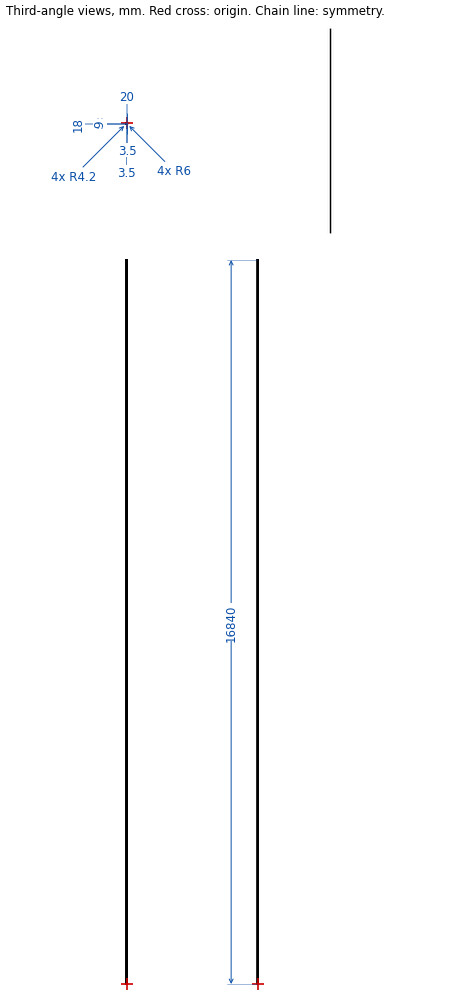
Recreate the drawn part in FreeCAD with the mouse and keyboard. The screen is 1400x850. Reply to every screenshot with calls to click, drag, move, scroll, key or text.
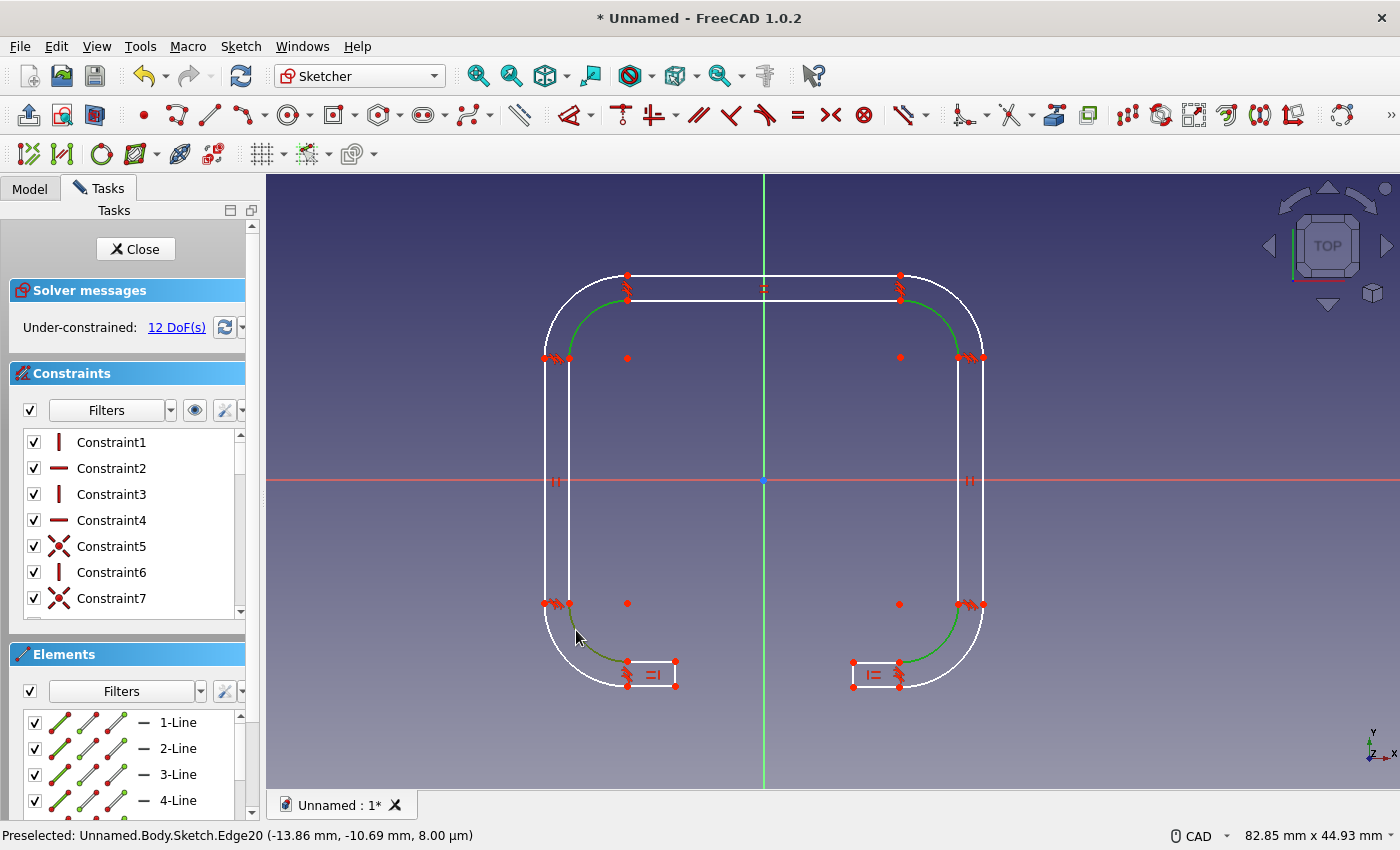
click(798, 116)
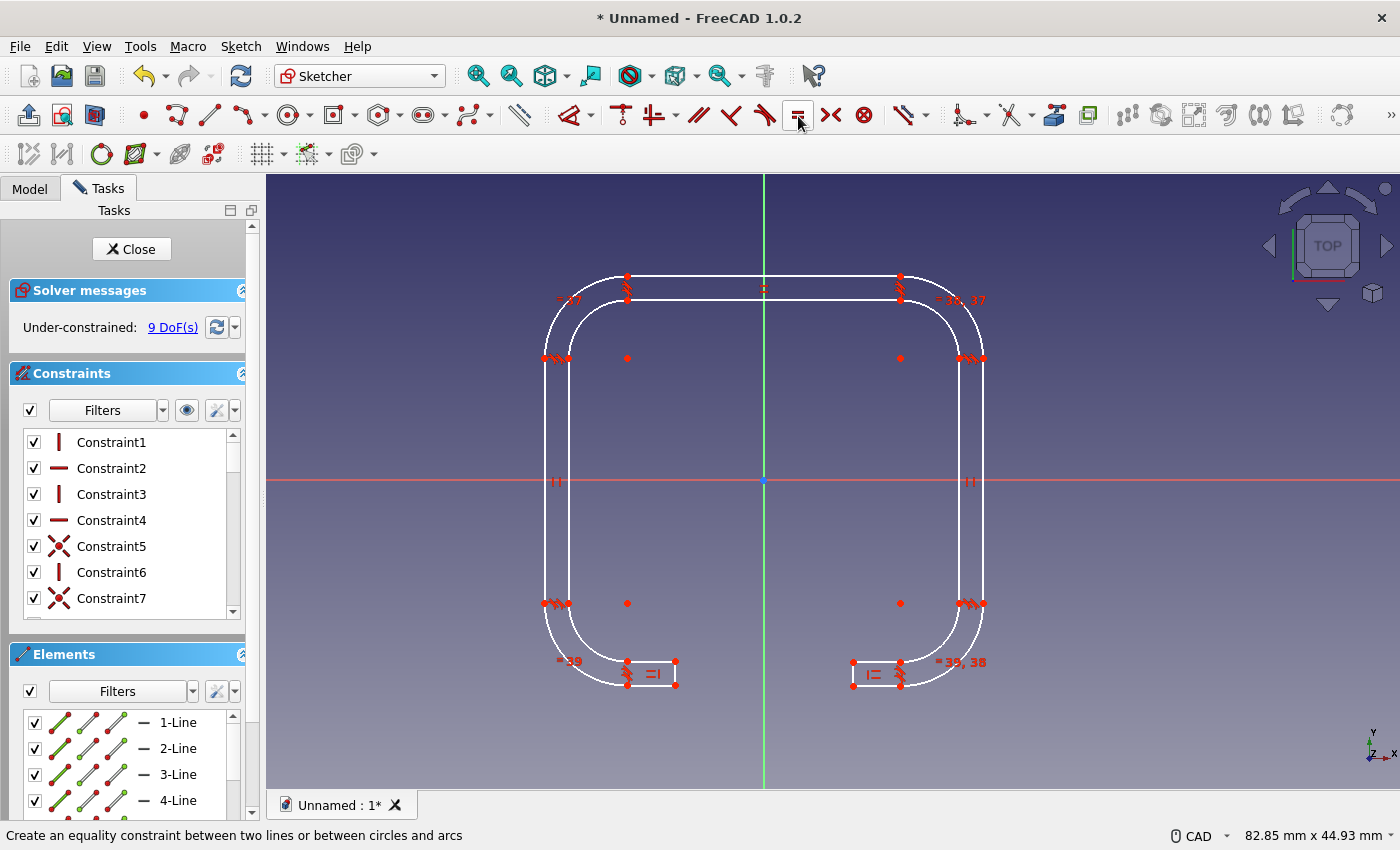
click(901, 604)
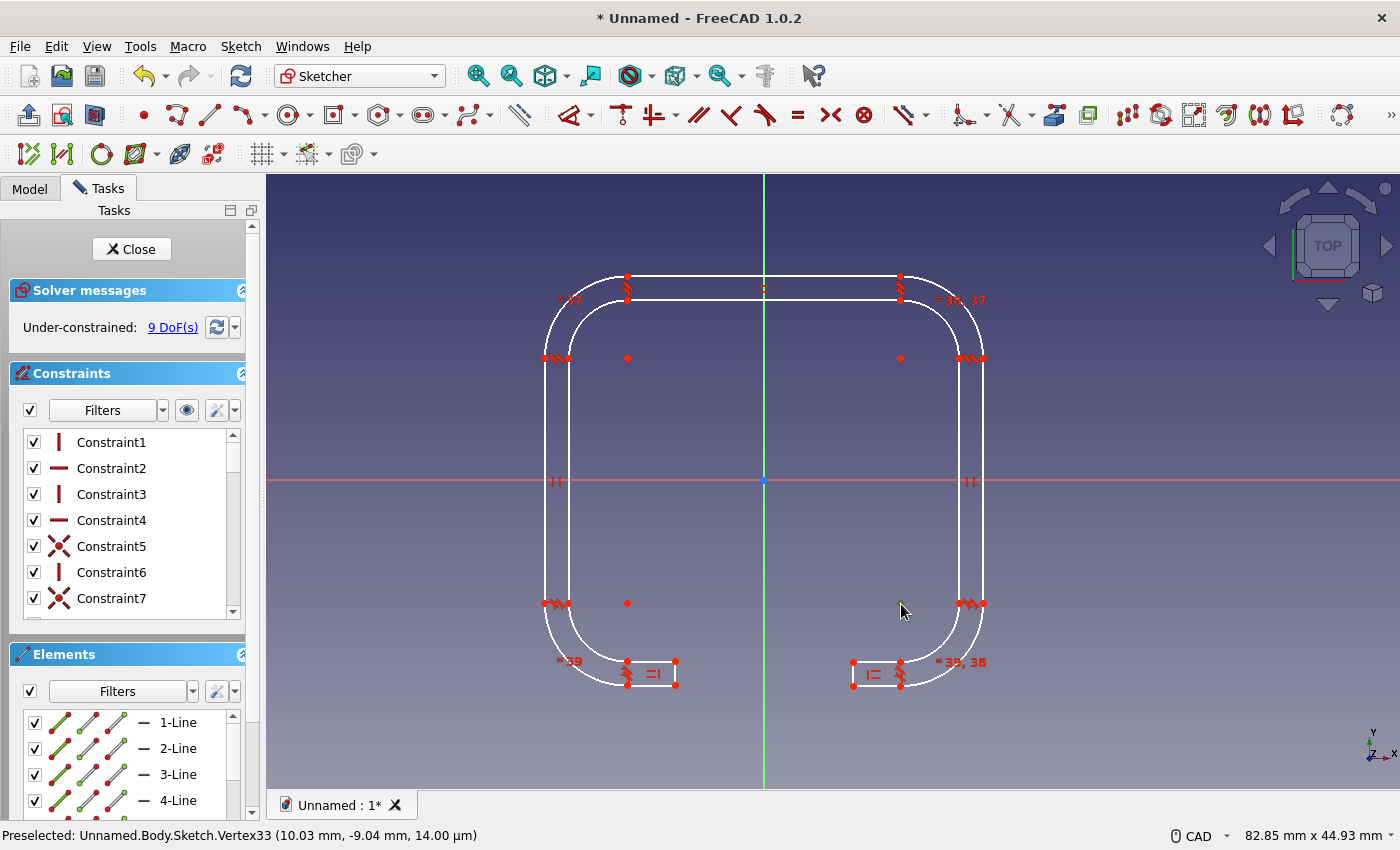
click(627, 603)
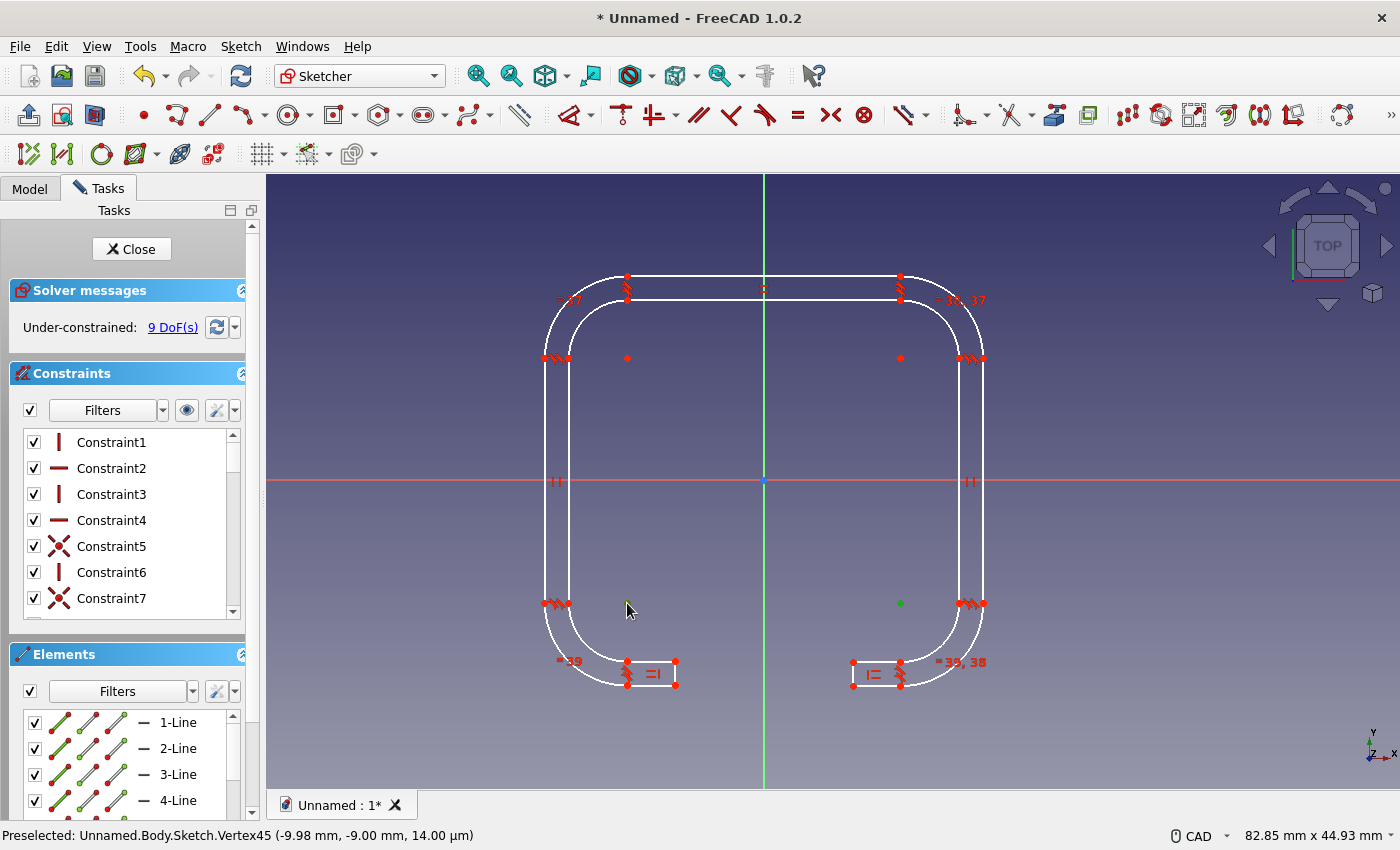
click(764, 721)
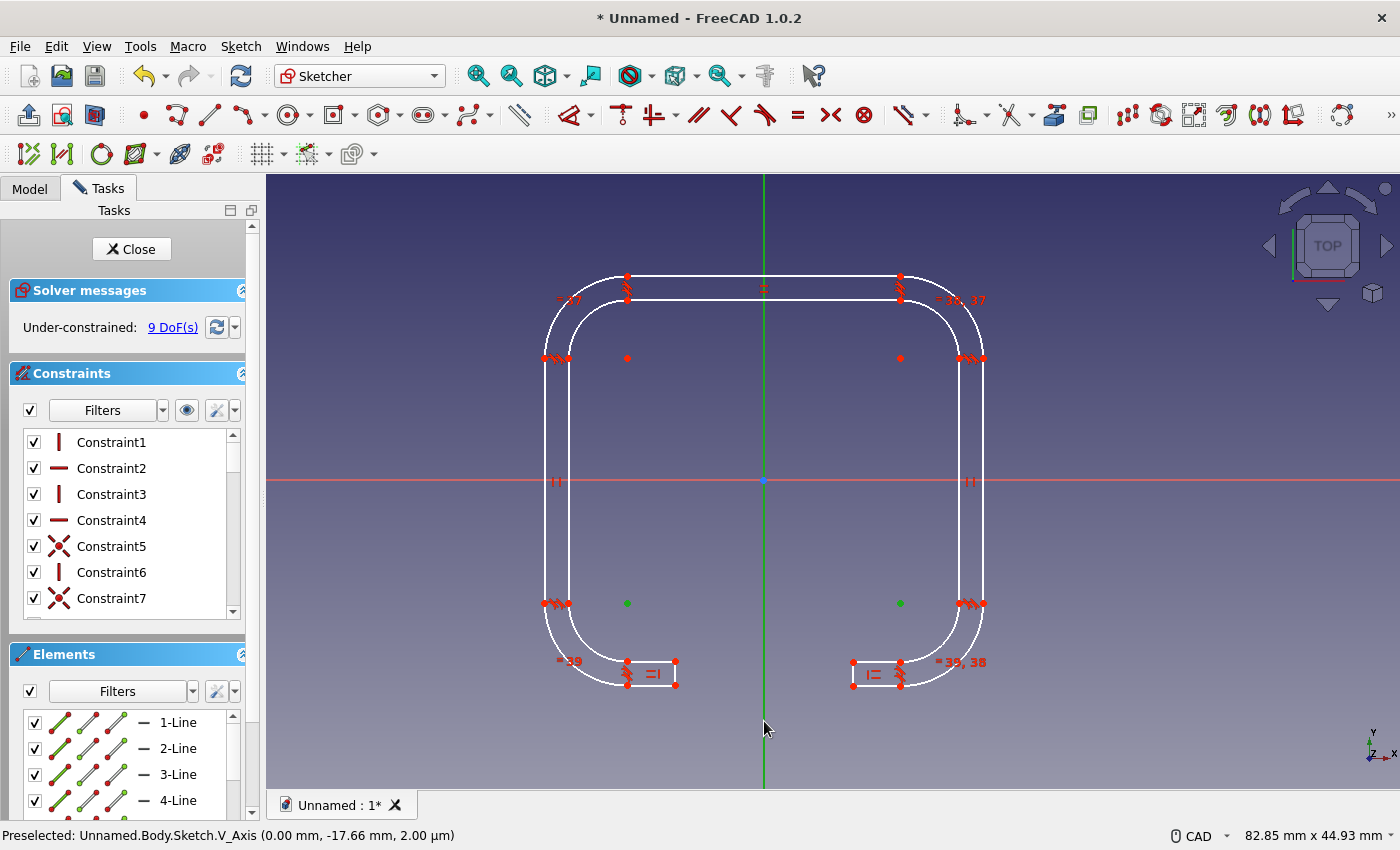
click(831, 116)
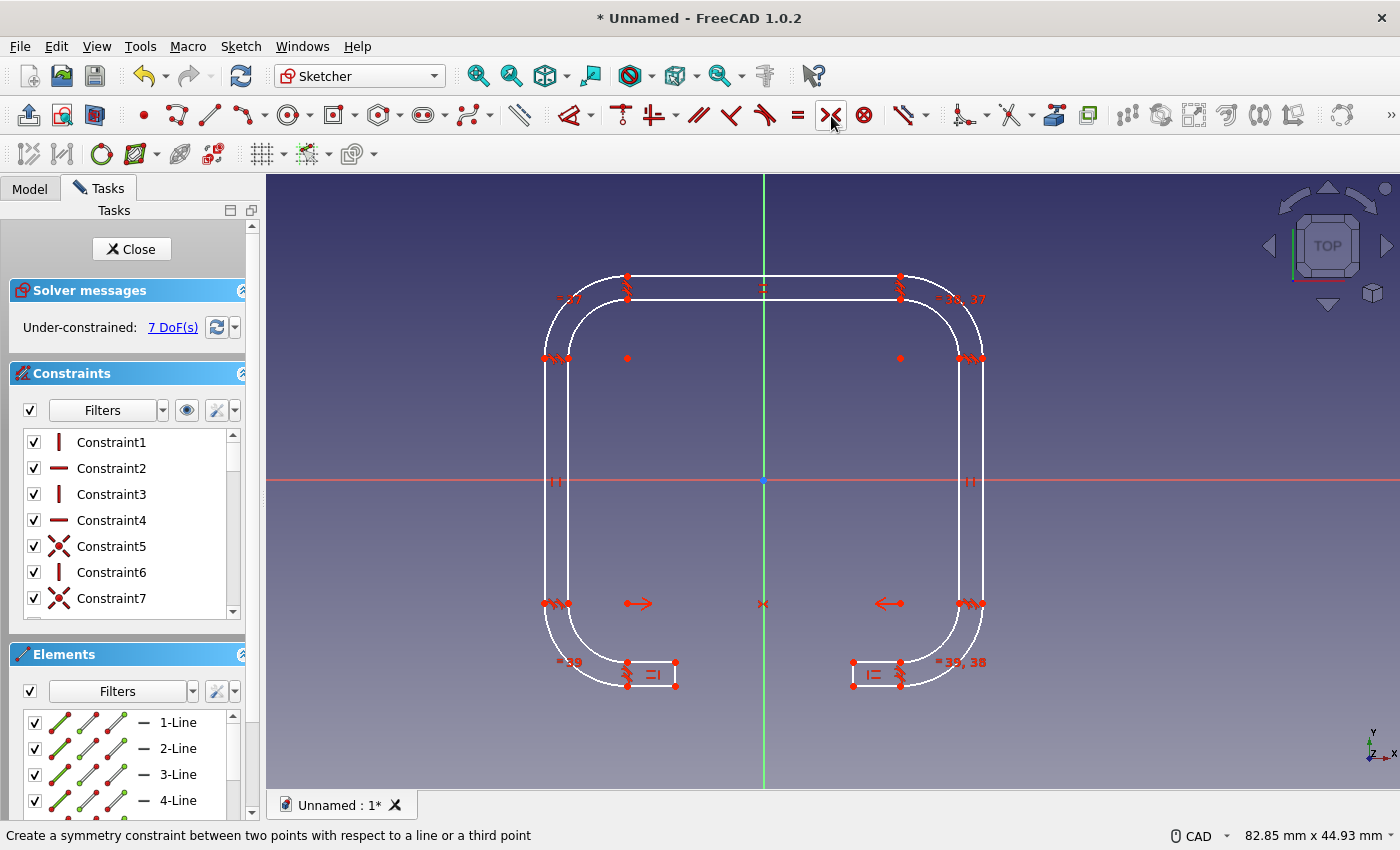
click(568, 116)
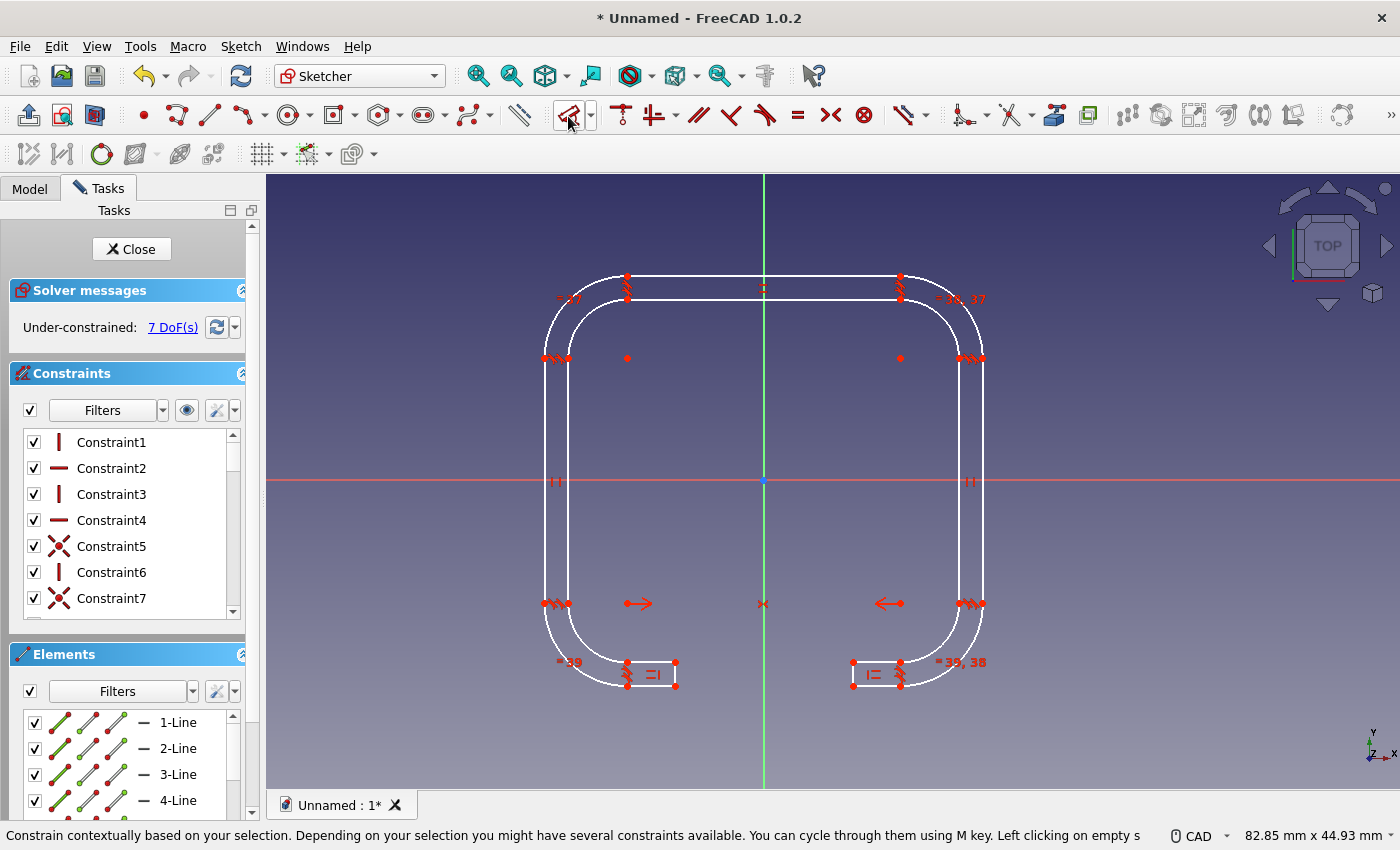
click(600, 306)
click(708, 317)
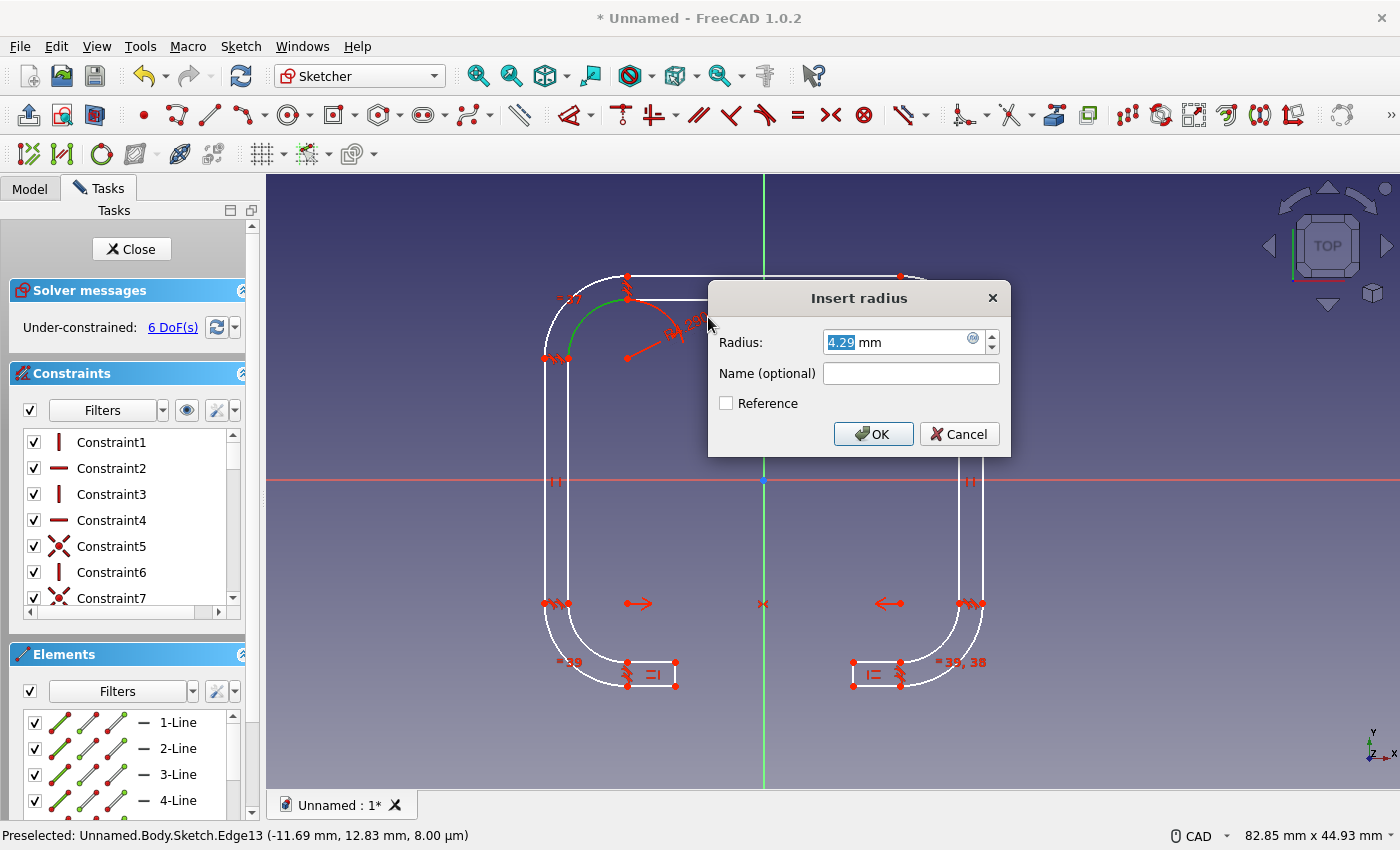
text(4.2)
key(Return)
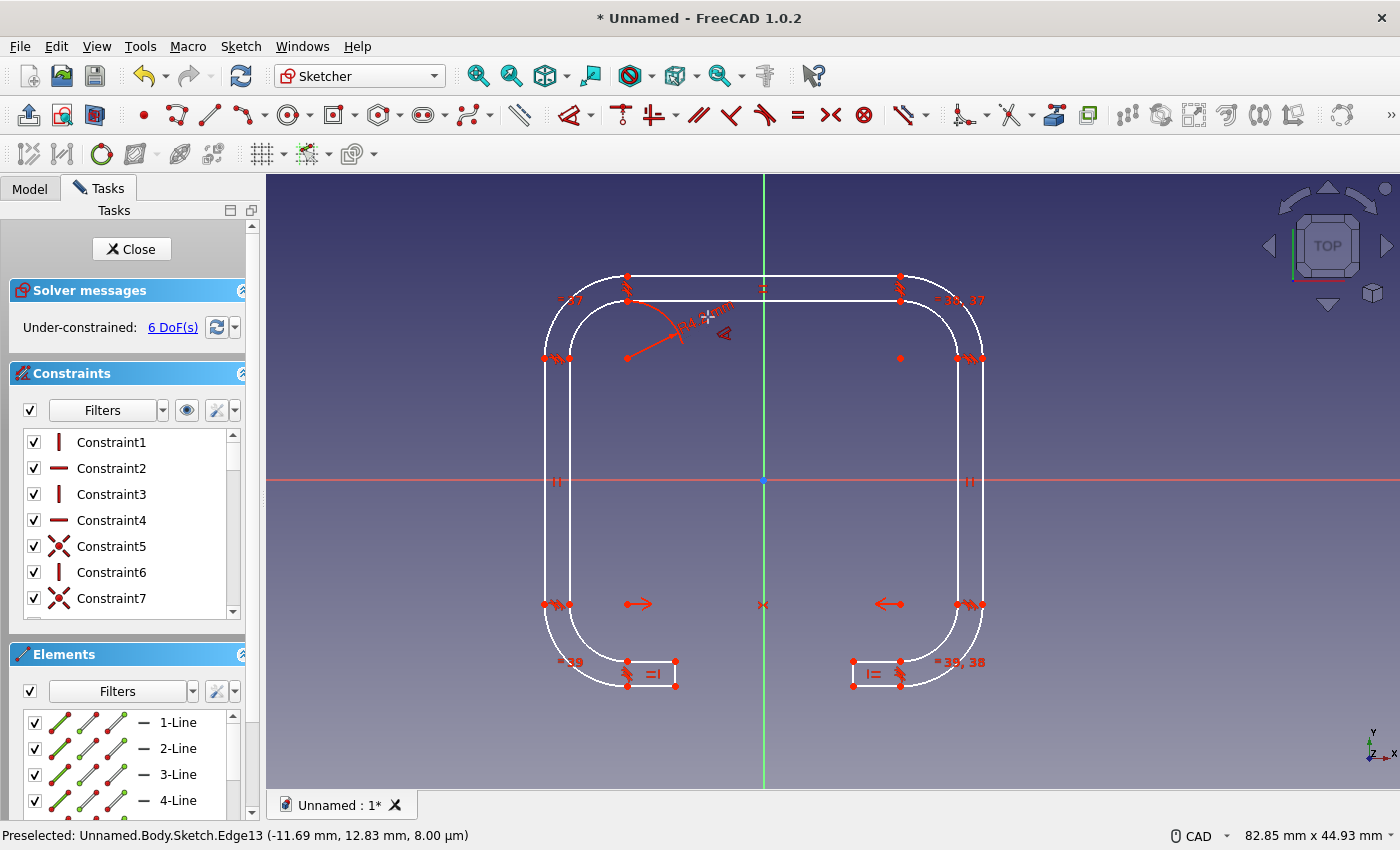
click(938, 677)
click(953, 705)